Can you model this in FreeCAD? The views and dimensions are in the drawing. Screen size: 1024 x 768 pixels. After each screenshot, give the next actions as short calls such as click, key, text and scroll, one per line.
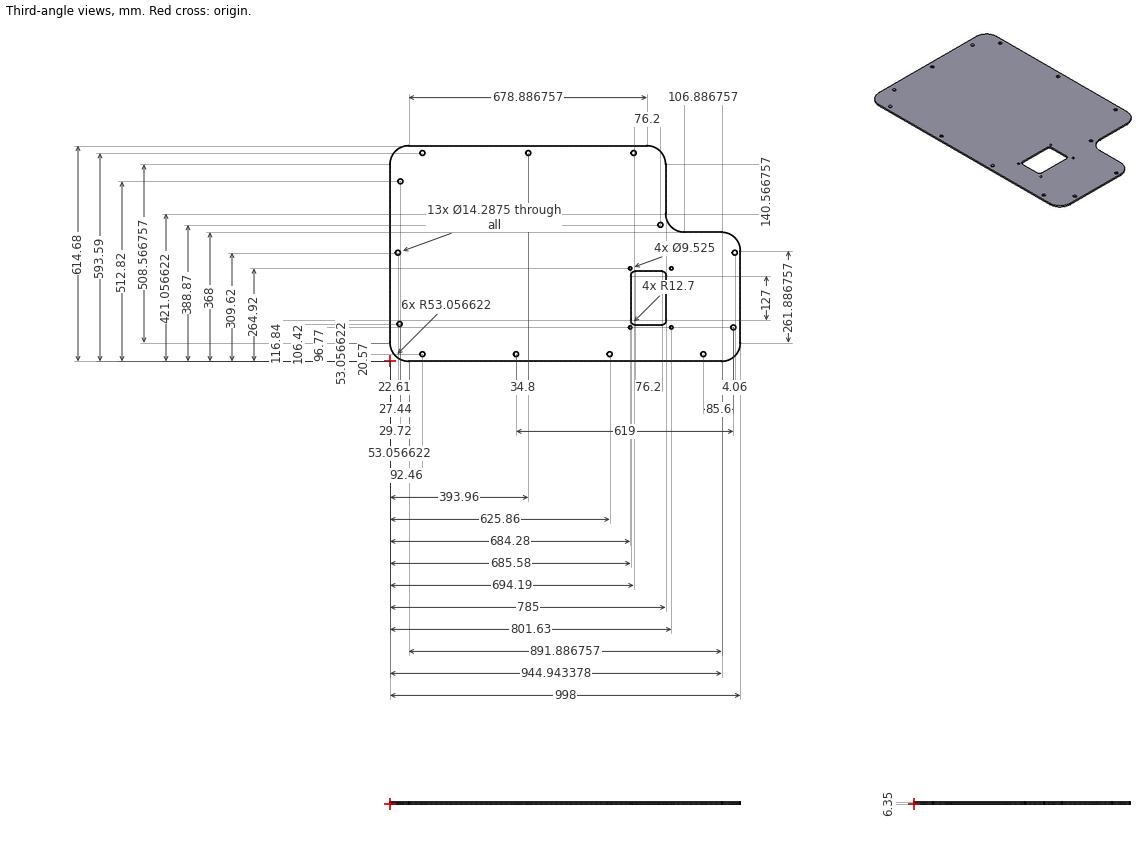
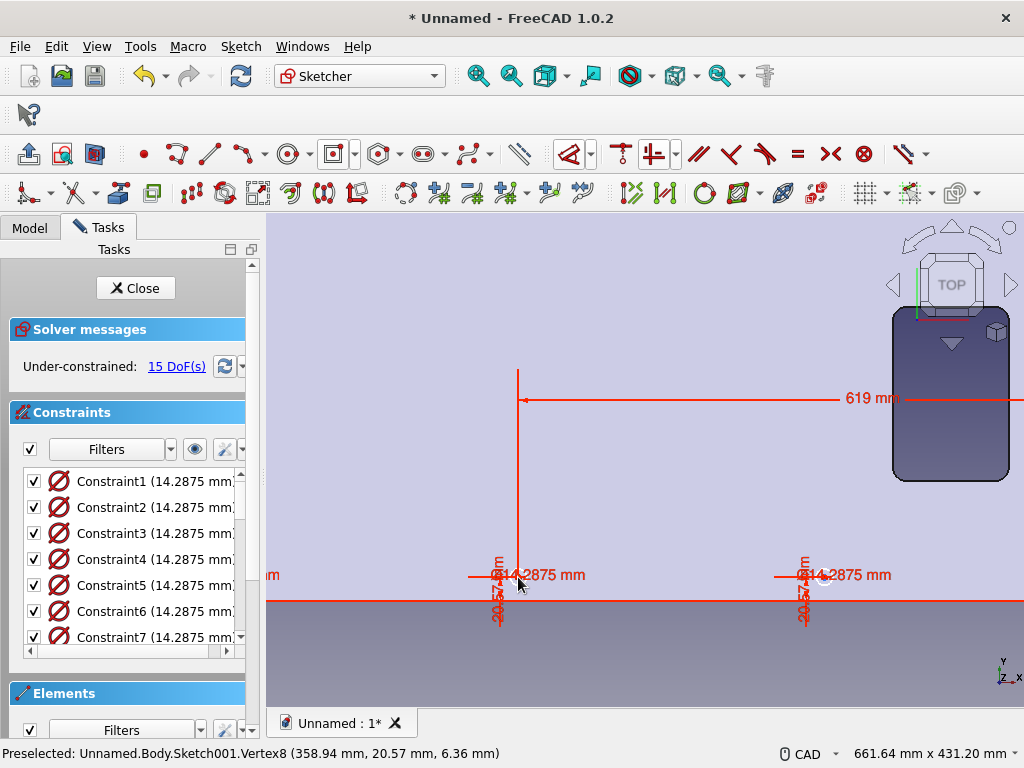
click(590, 154)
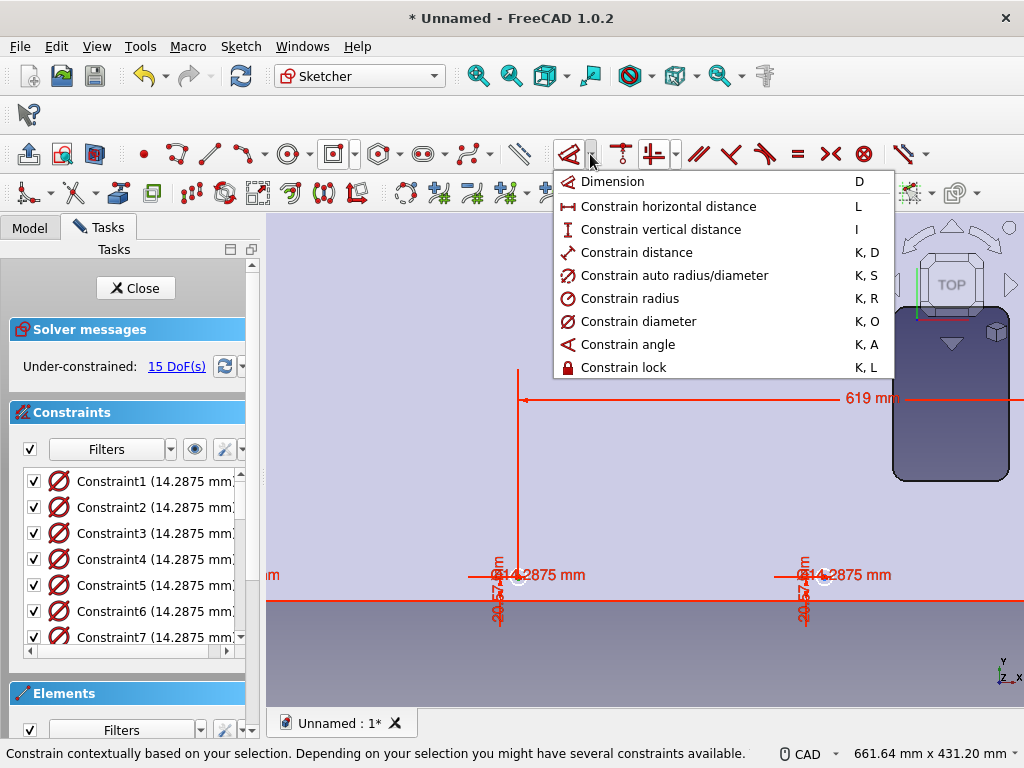
click(724, 206)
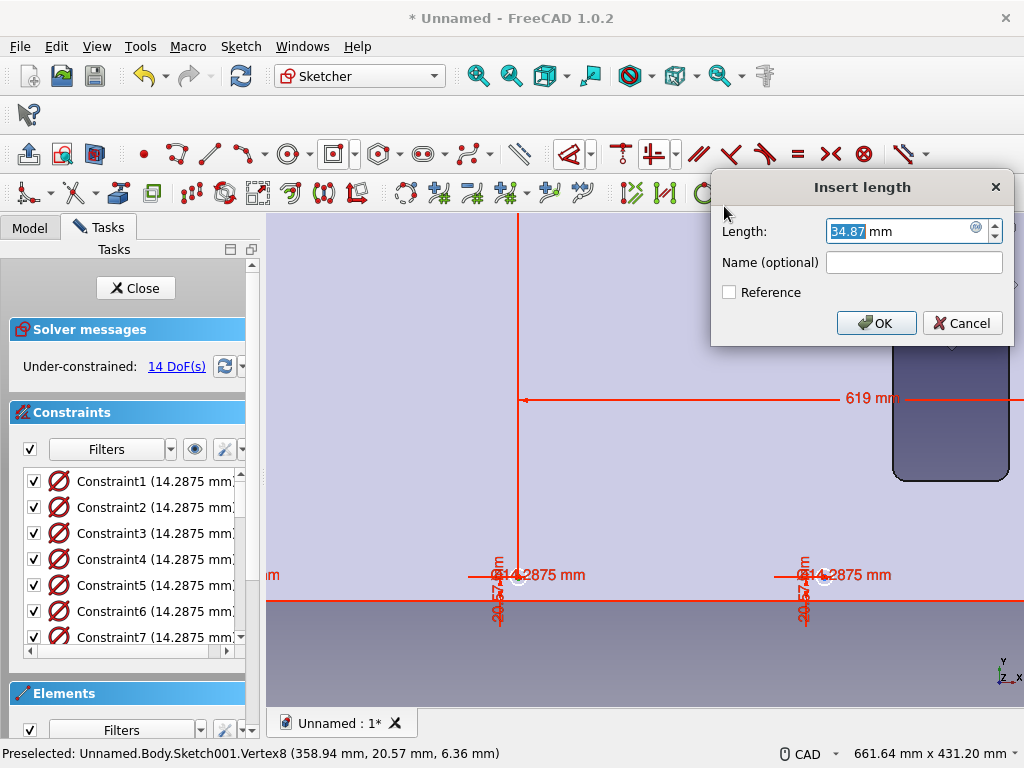
text(34.8)
key(Return)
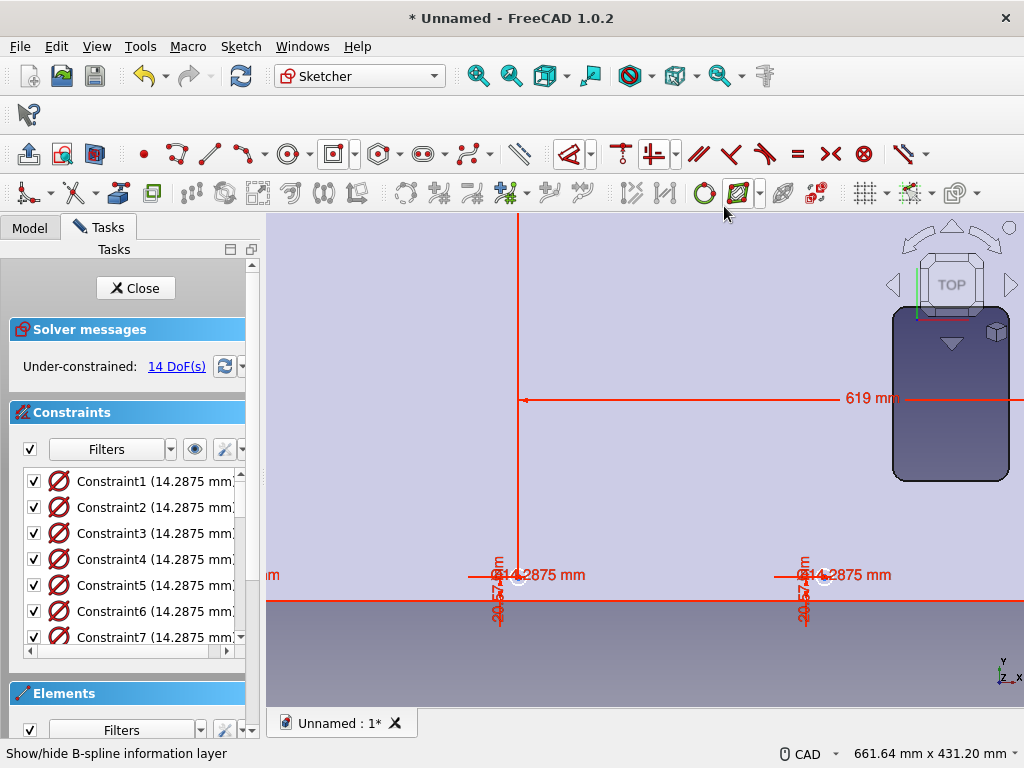
scroll(520, 578, down, 5)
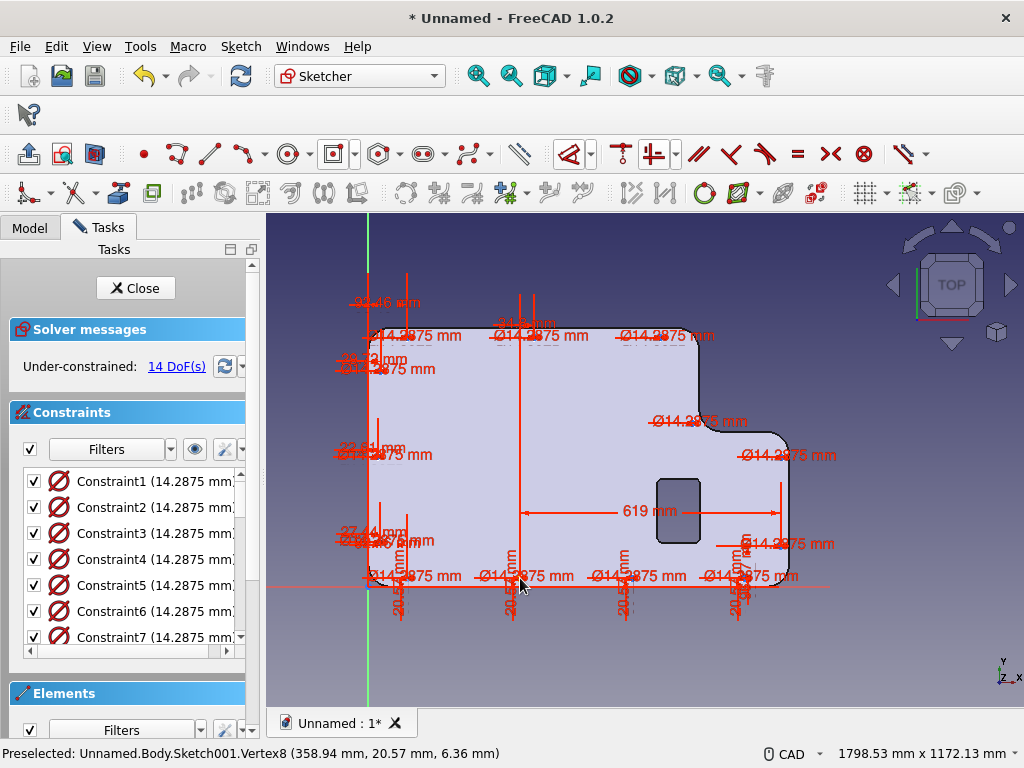
click(744, 578)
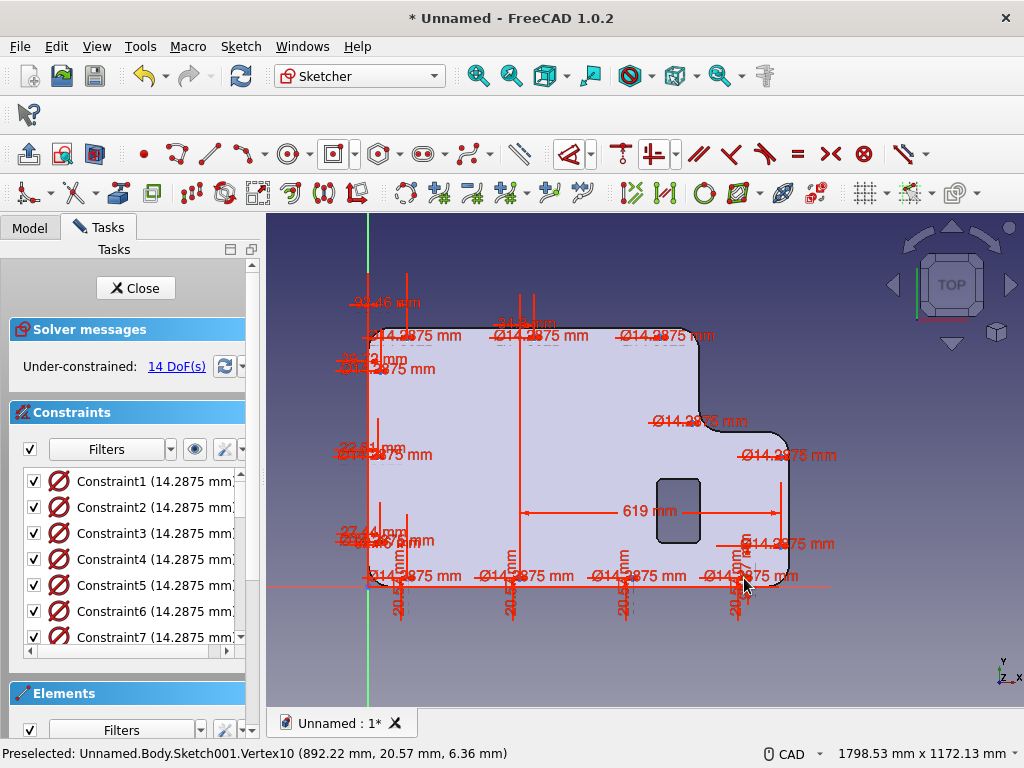
click(781, 546)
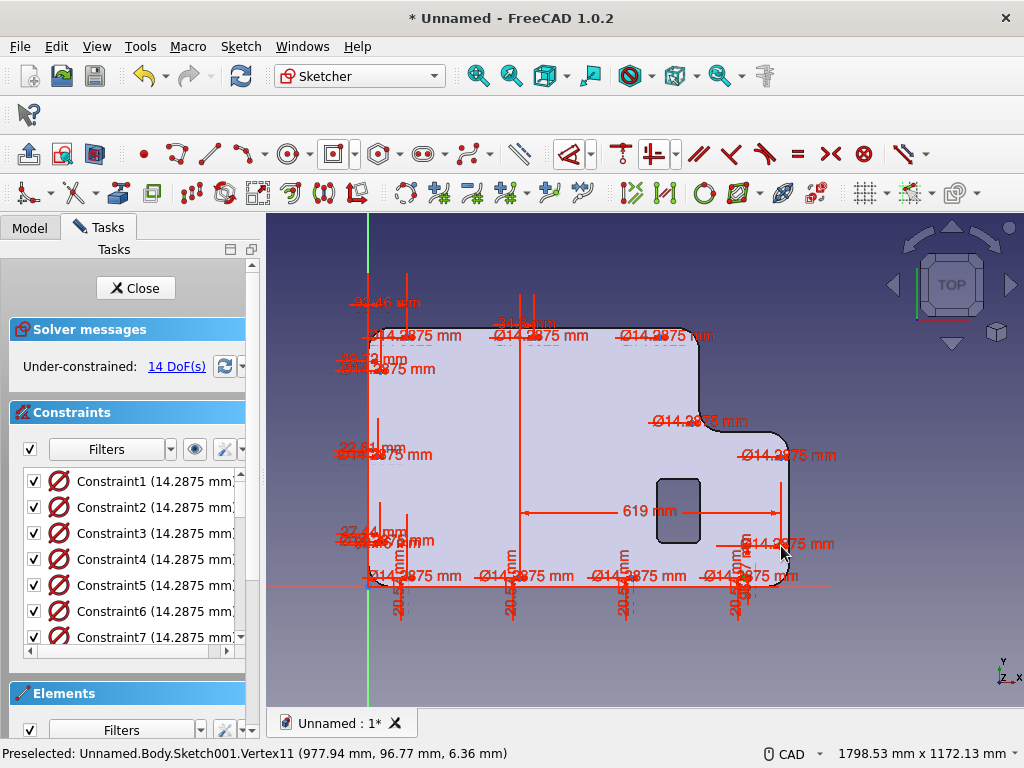
click(590, 154)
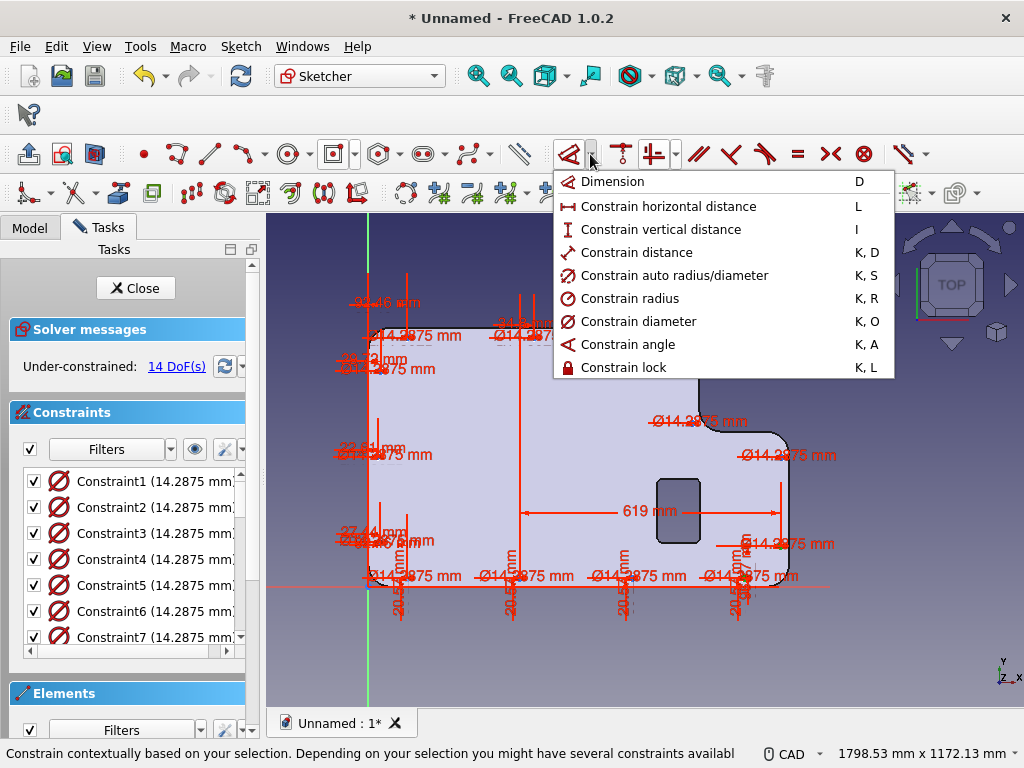
click(724, 206)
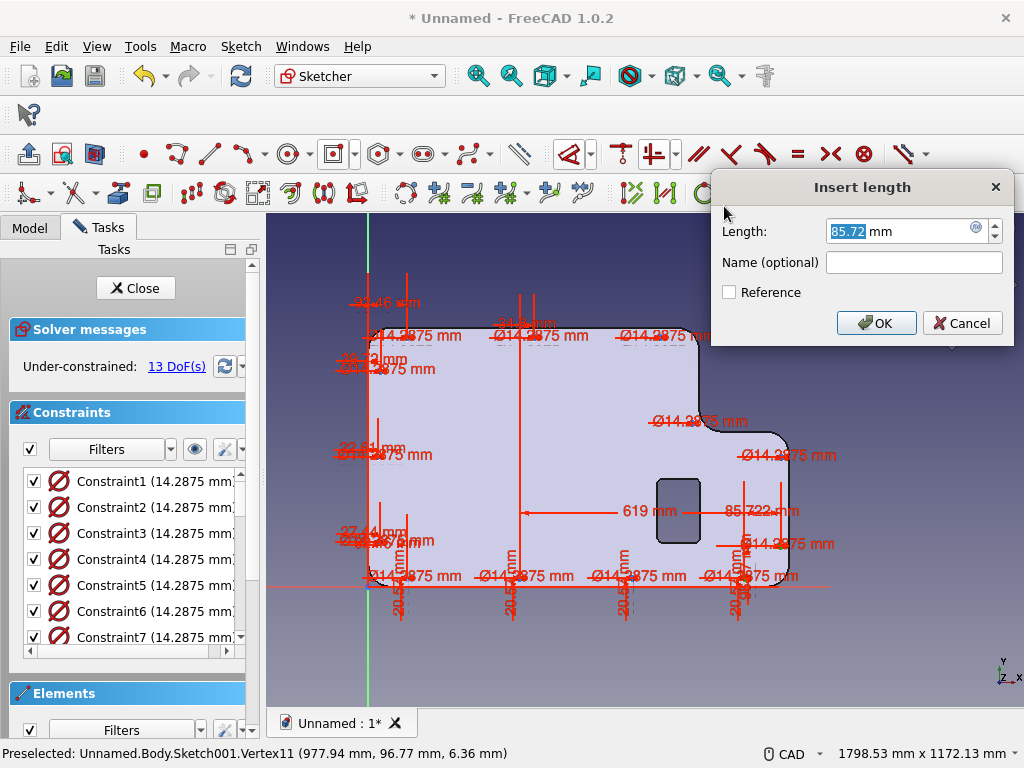
text(85.6)
key(Return)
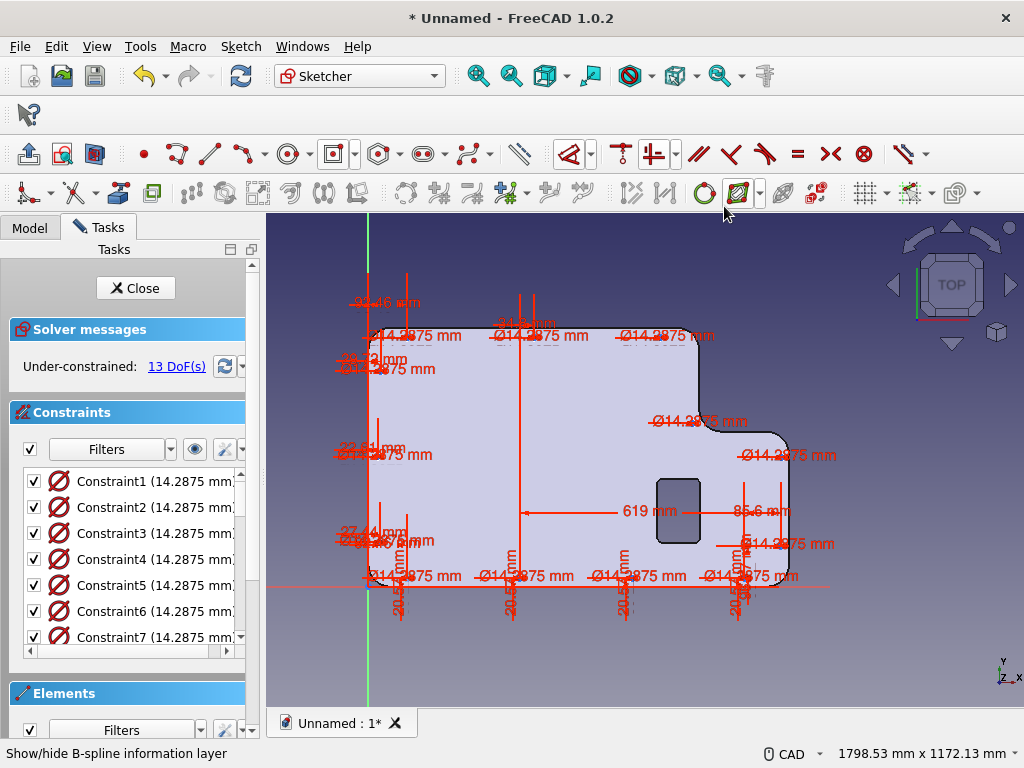
scroll(781, 546, up, 16)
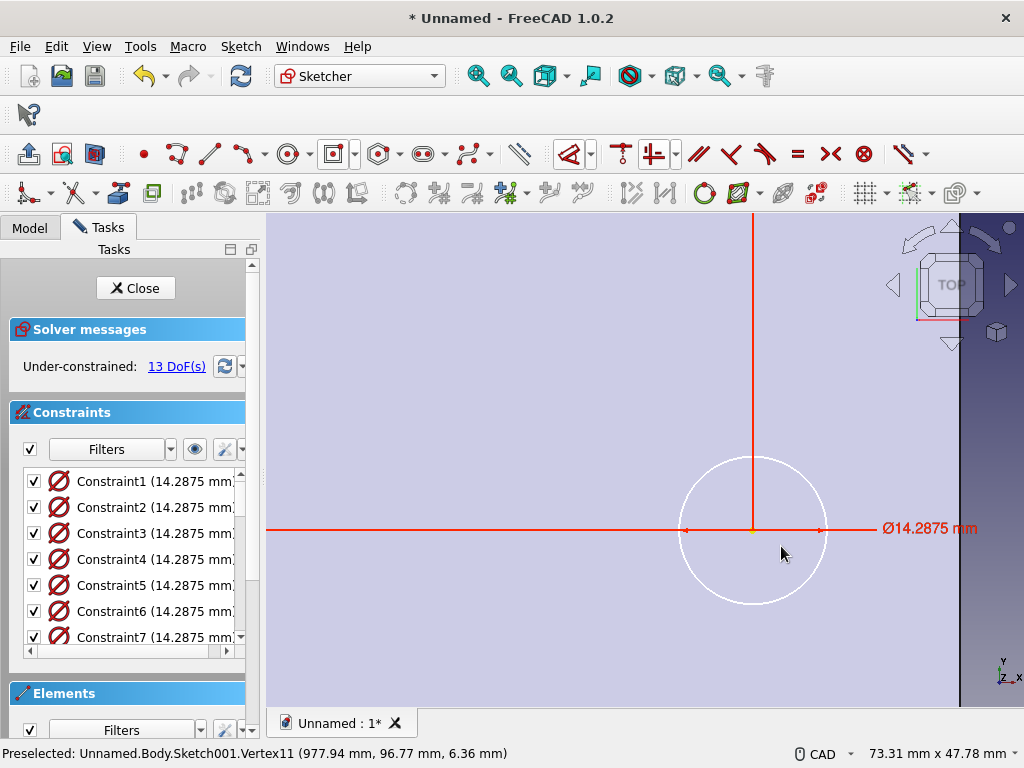
click(753, 530)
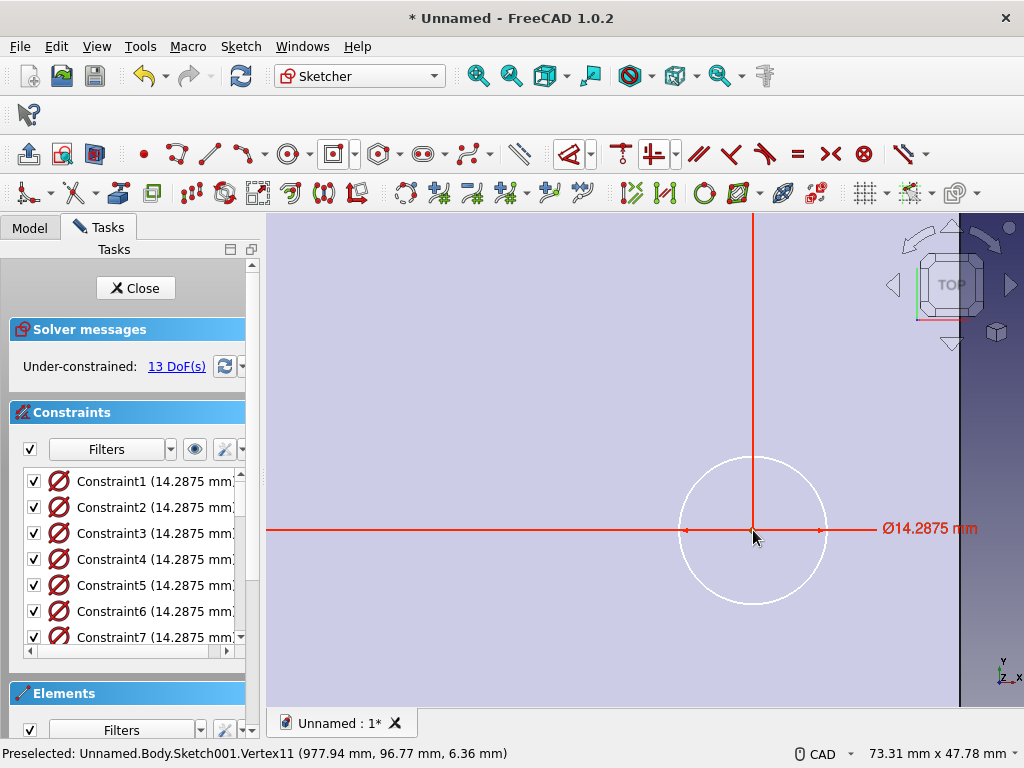
scroll(829, 567, down, 15)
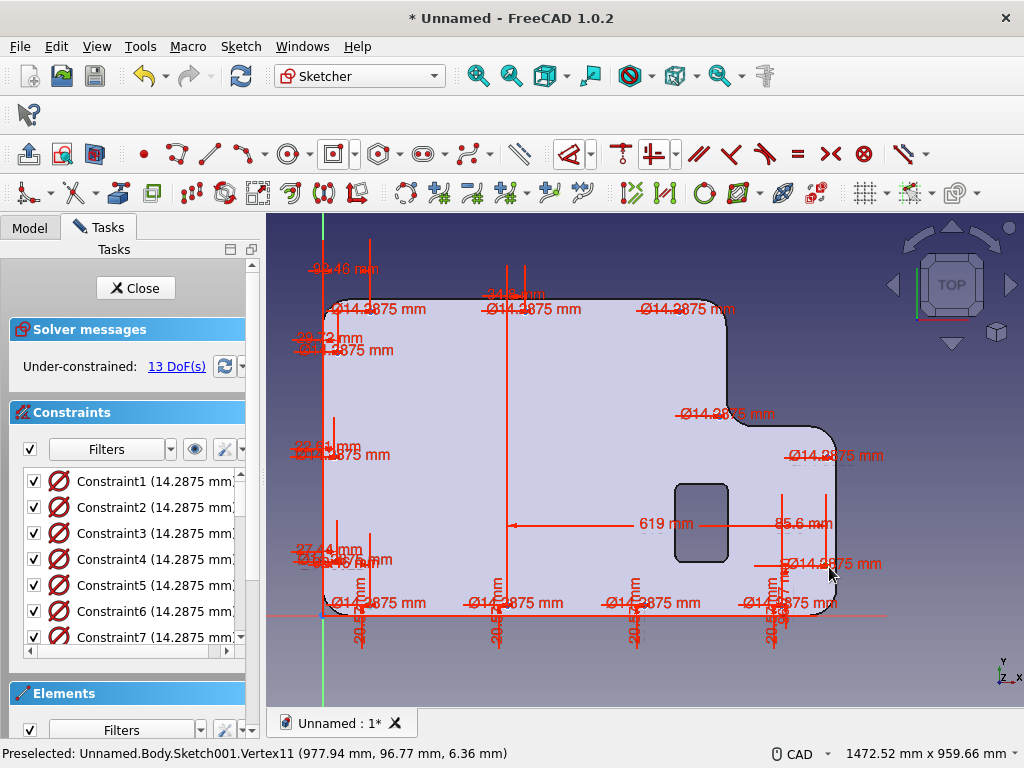
scroll(828, 458, up, 15)